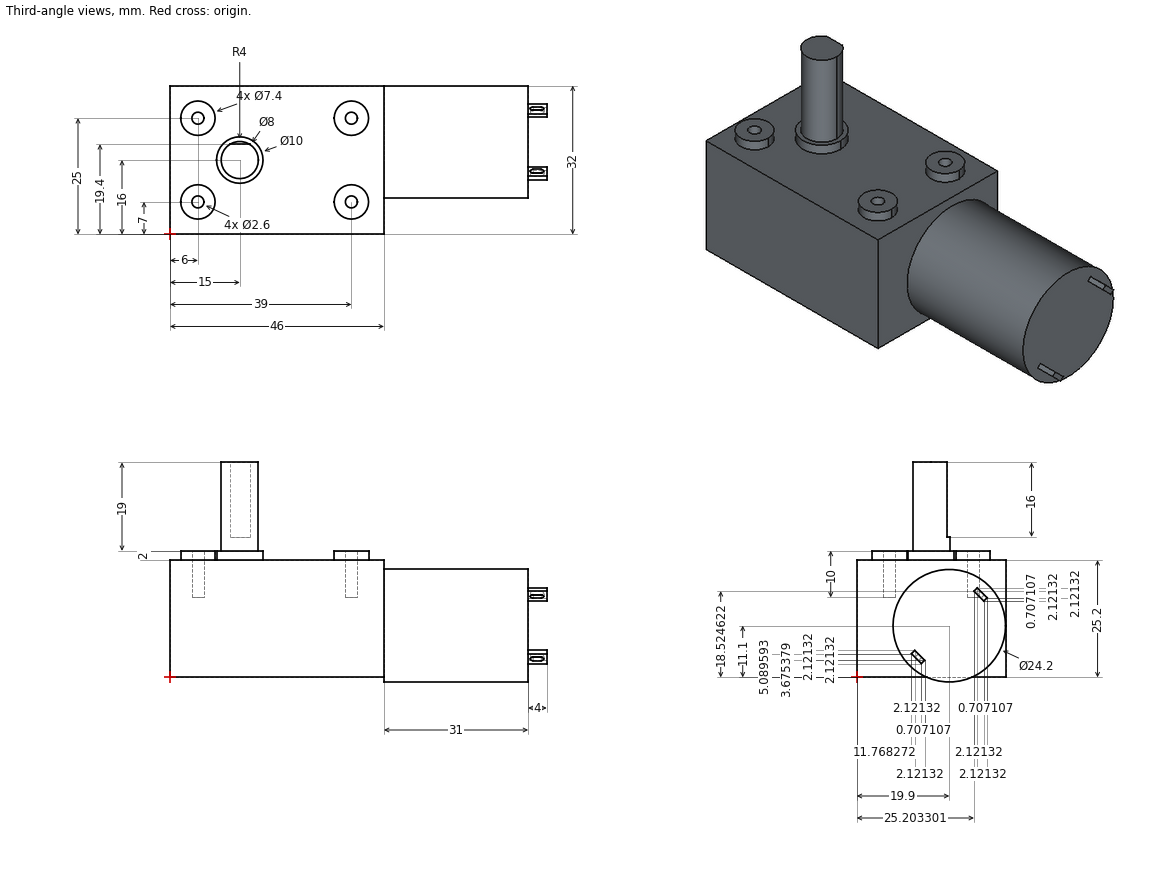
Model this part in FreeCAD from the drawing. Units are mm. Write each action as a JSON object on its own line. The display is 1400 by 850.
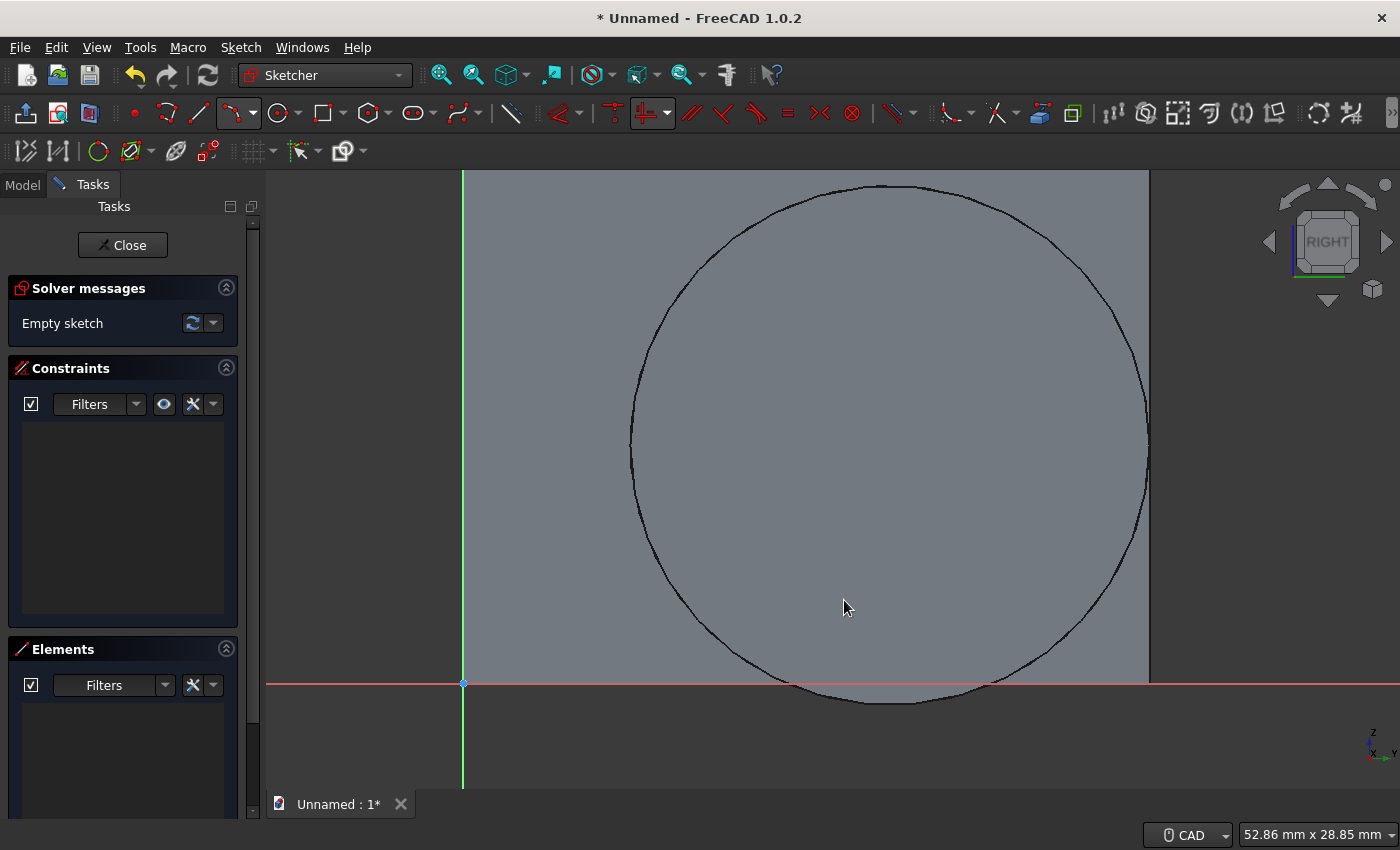
{"action": "left_click", "coordinate": [168, 114]}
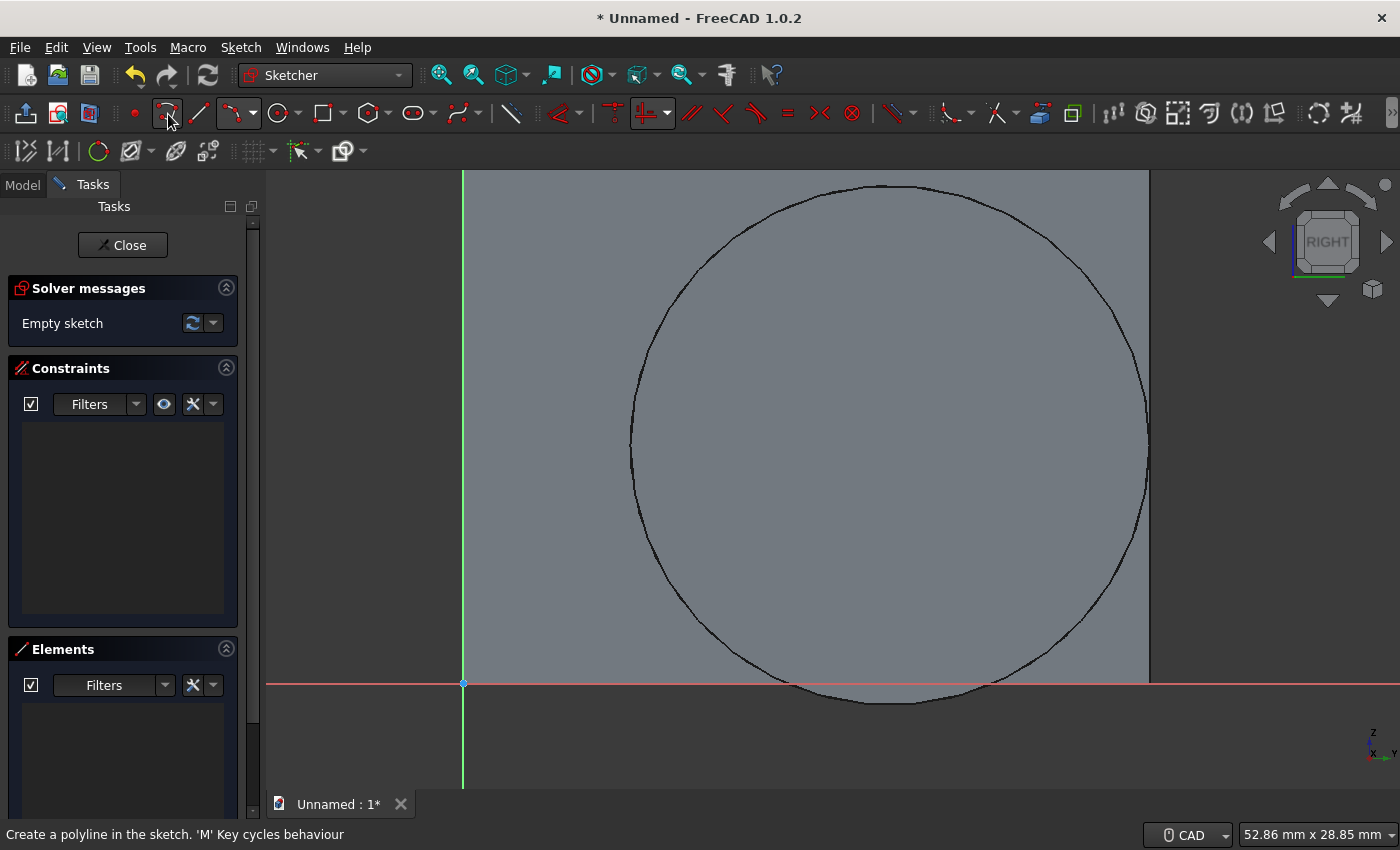
{"action": "left_click", "coordinate": [1004, 286]}
{"action": "left_click", "coordinate": [1049, 332]}
{"action": "left_click", "coordinate": [1064, 317]}
{"action": "left_click", "coordinate": [1019, 271]}
{"action": "left_click", "coordinate": [1004, 287]}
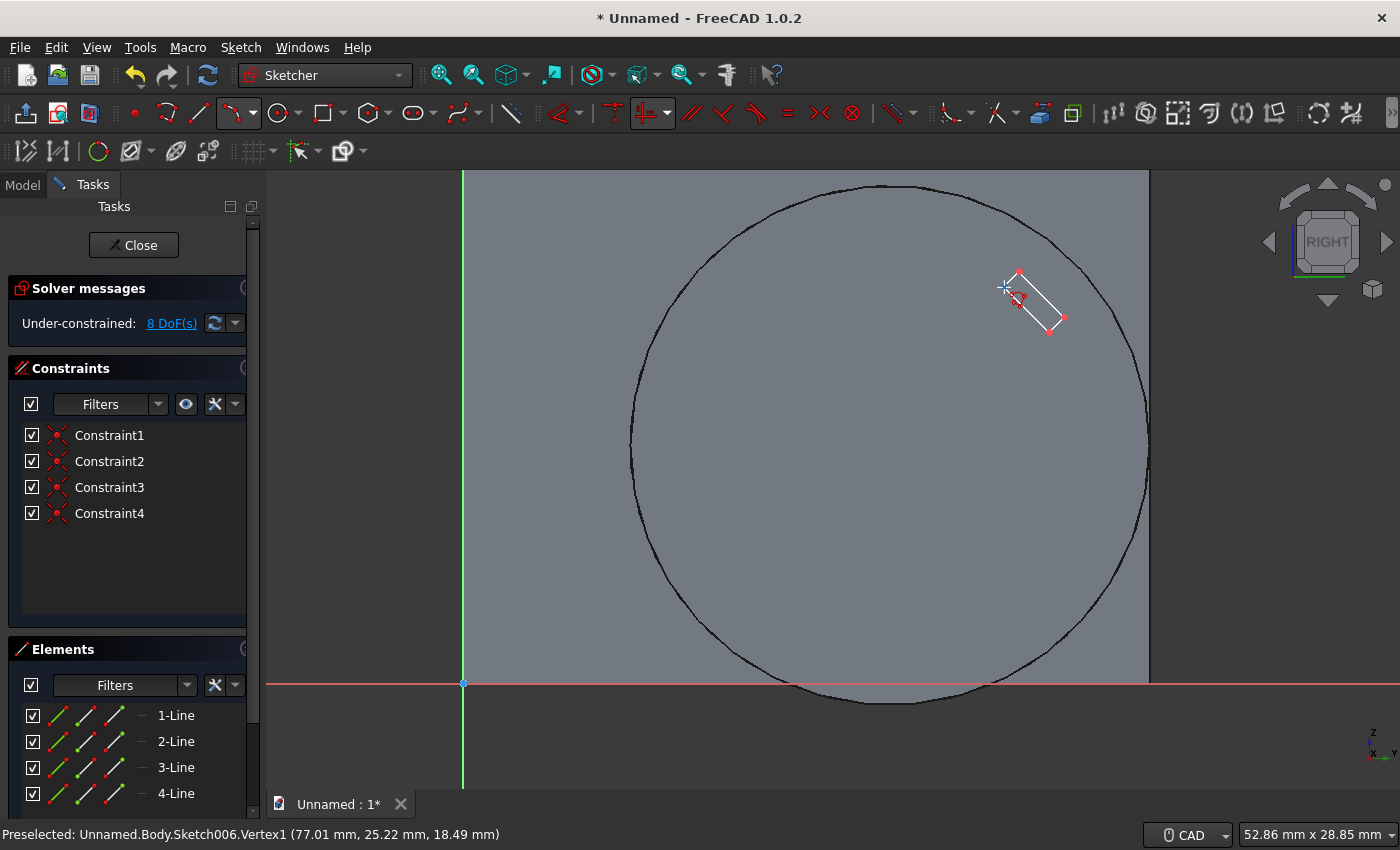
{"action": "left_click", "coordinate": [716, 574]}
{"action": "left_click", "coordinate": [761, 620]}
{"action": "left_click", "coordinate": [776, 605]}
{"action": "left_click", "coordinate": [731, 559]}
{"action": "left_click", "coordinate": [716, 575]}
{"action": "key", "text": "Escape"}
{"action": "key", "text": "Escape"}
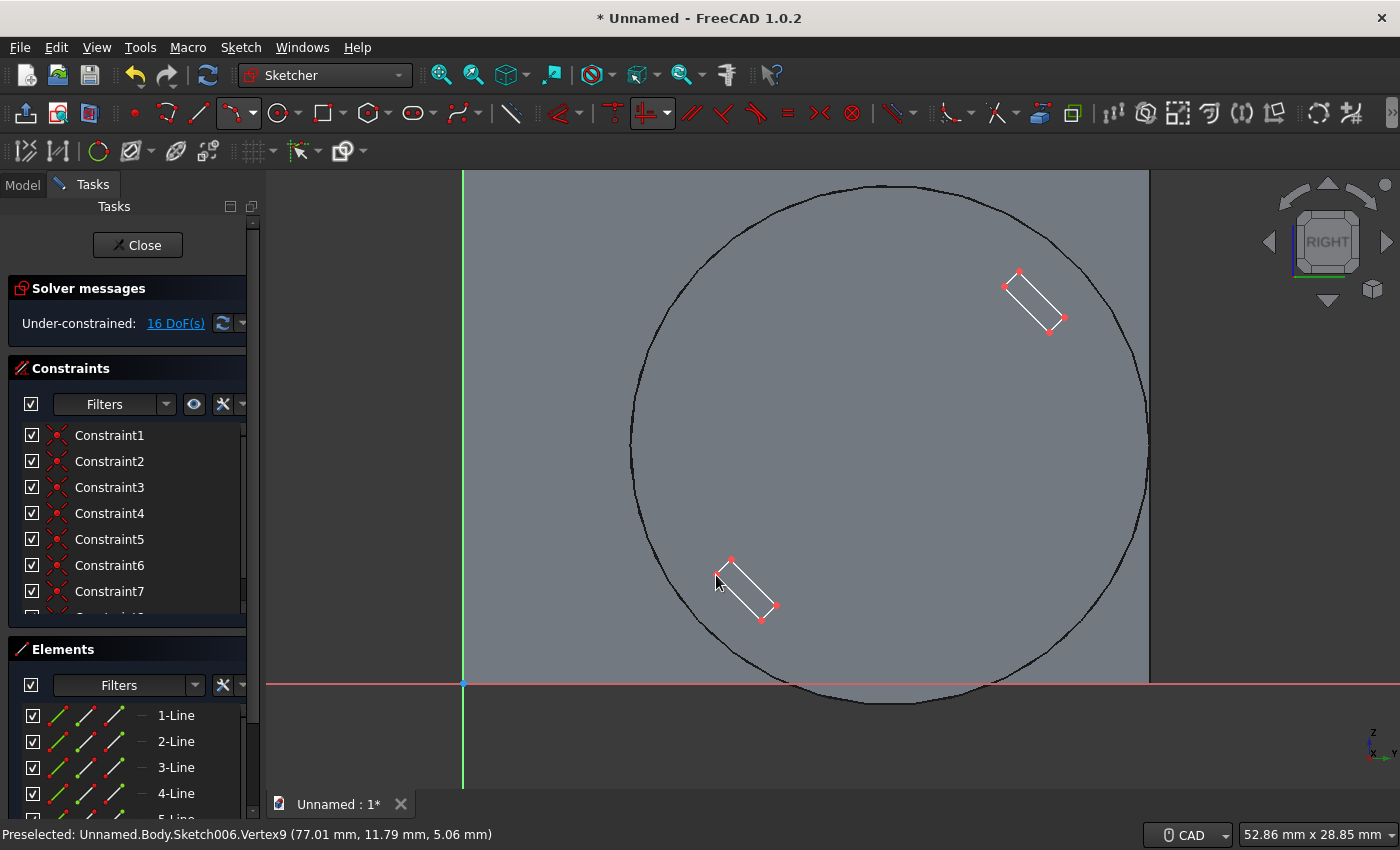
{"action": "key", "text": "d"}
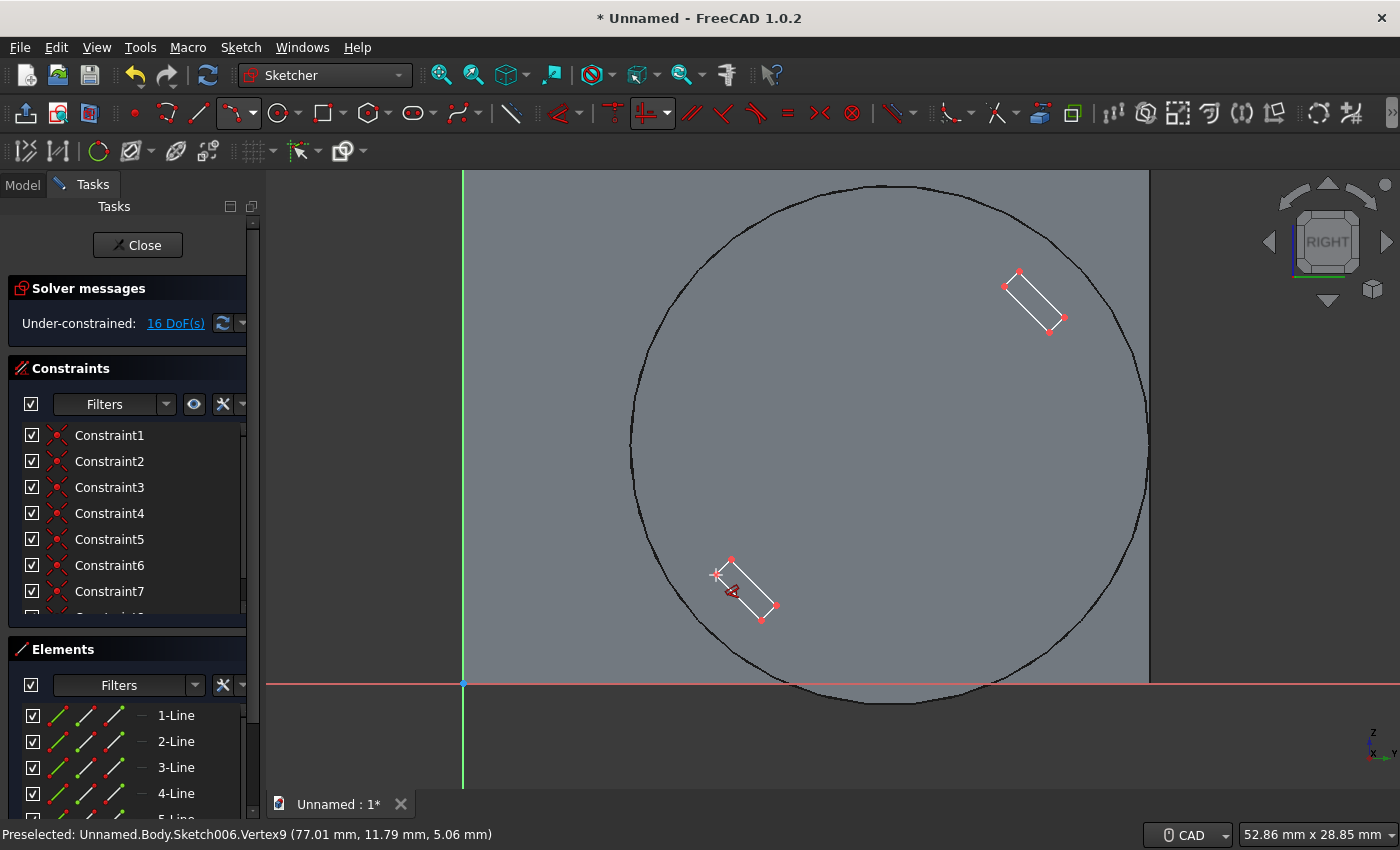
{"action": "left_click", "coordinate": [1018, 301]}
{"action": "left_click", "coordinate": [1027, 253]}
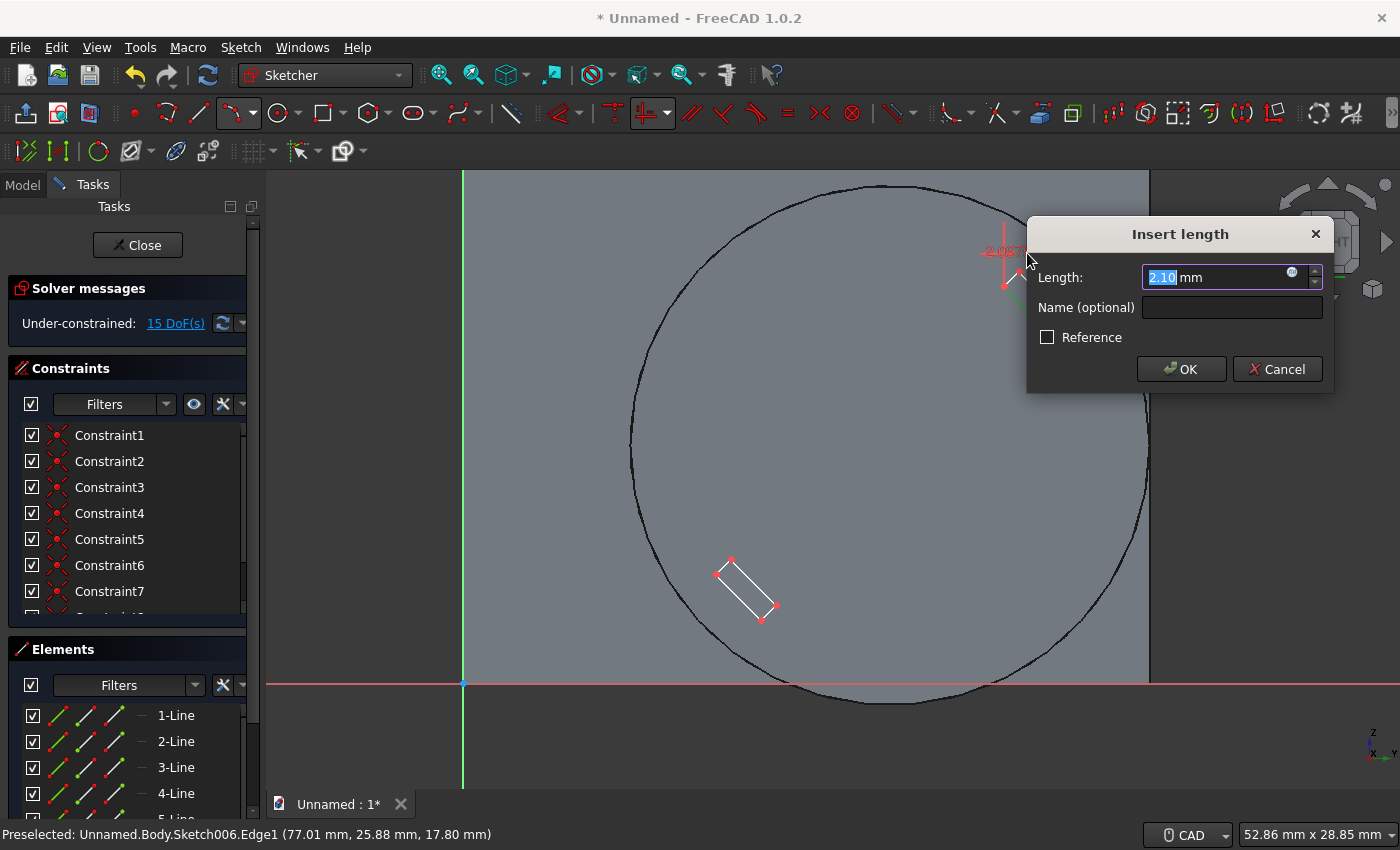
{"action": "type", "text": "2.12132"}
{"action": "key", "text": "Return"}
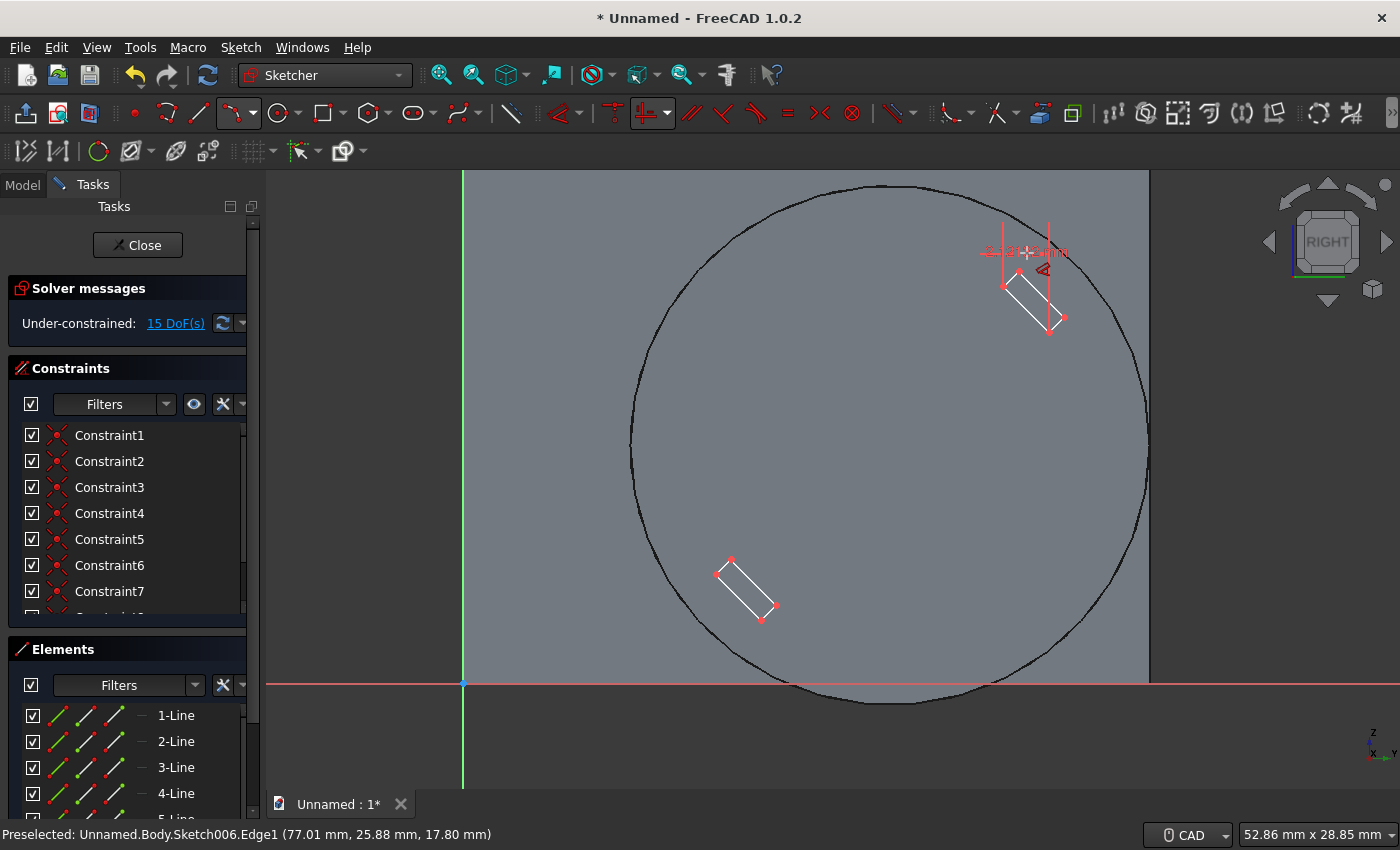
{"action": "left_click", "coordinate": [1017, 301]}
{"action": "left_click", "coordinate": [1083, 310]}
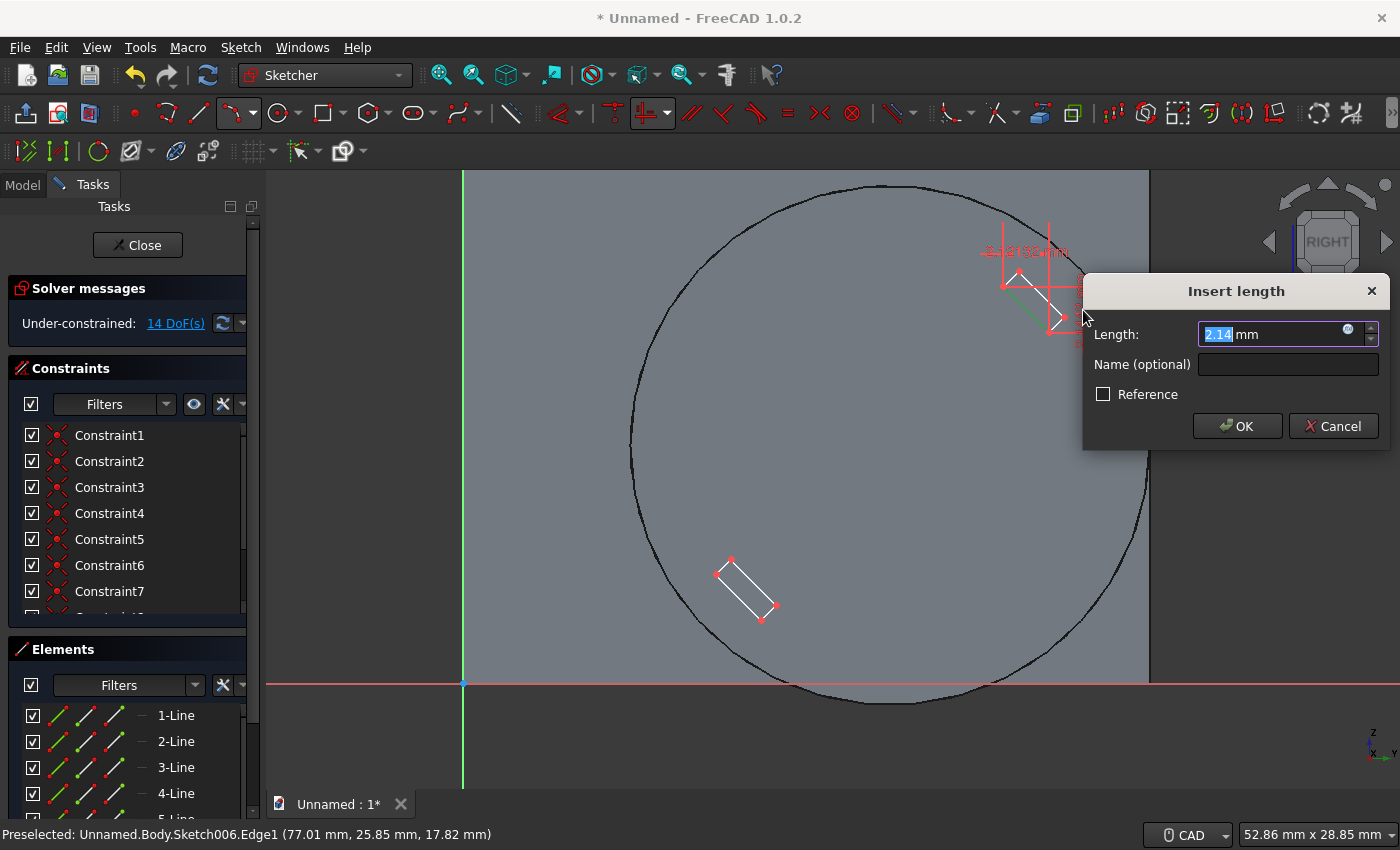
{"action": "type", "text": "2.12132"}
{"action": "key", "text": "Return"}